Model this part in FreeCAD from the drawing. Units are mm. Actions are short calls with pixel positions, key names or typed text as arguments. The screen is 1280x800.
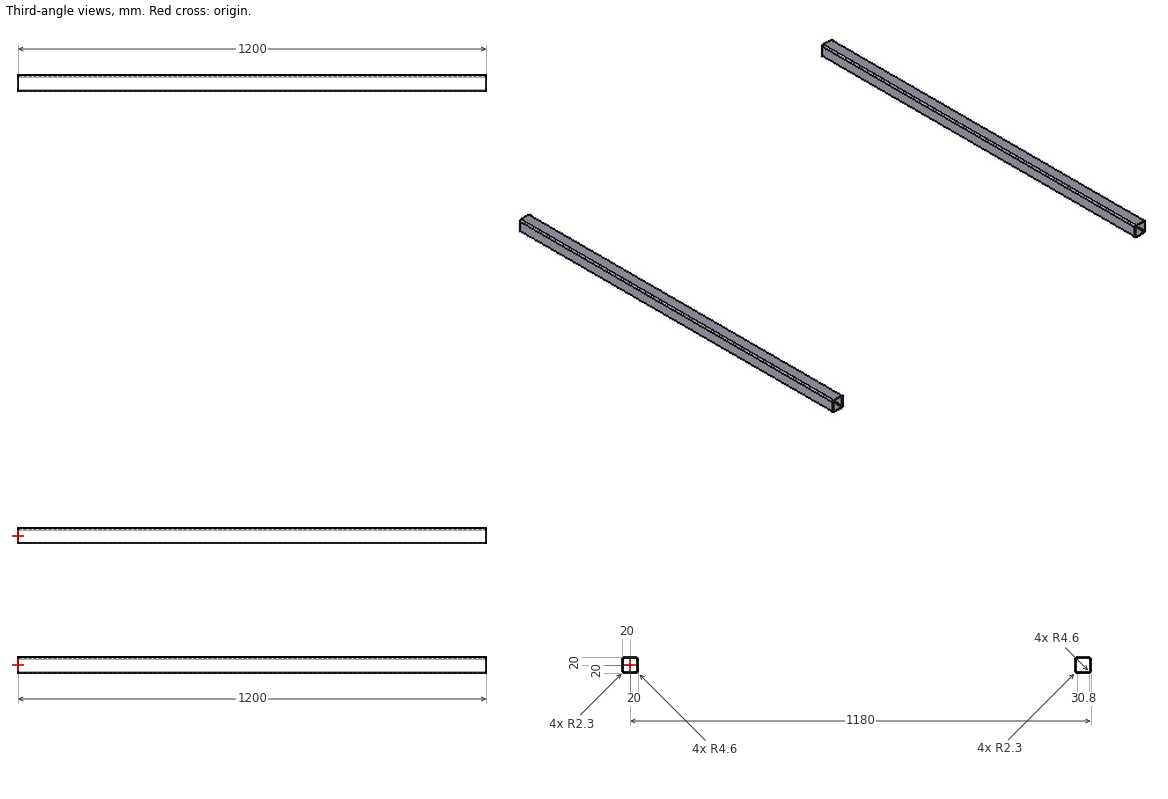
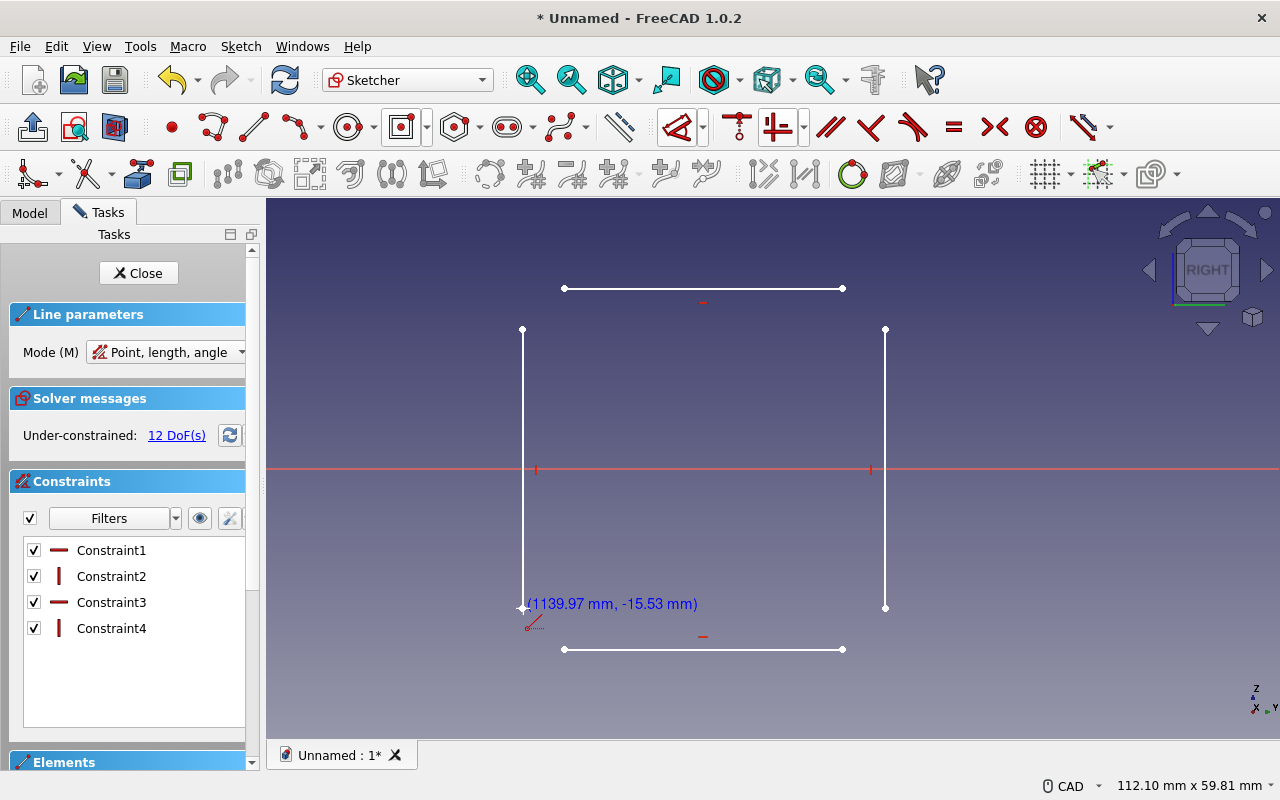
click(294, 128)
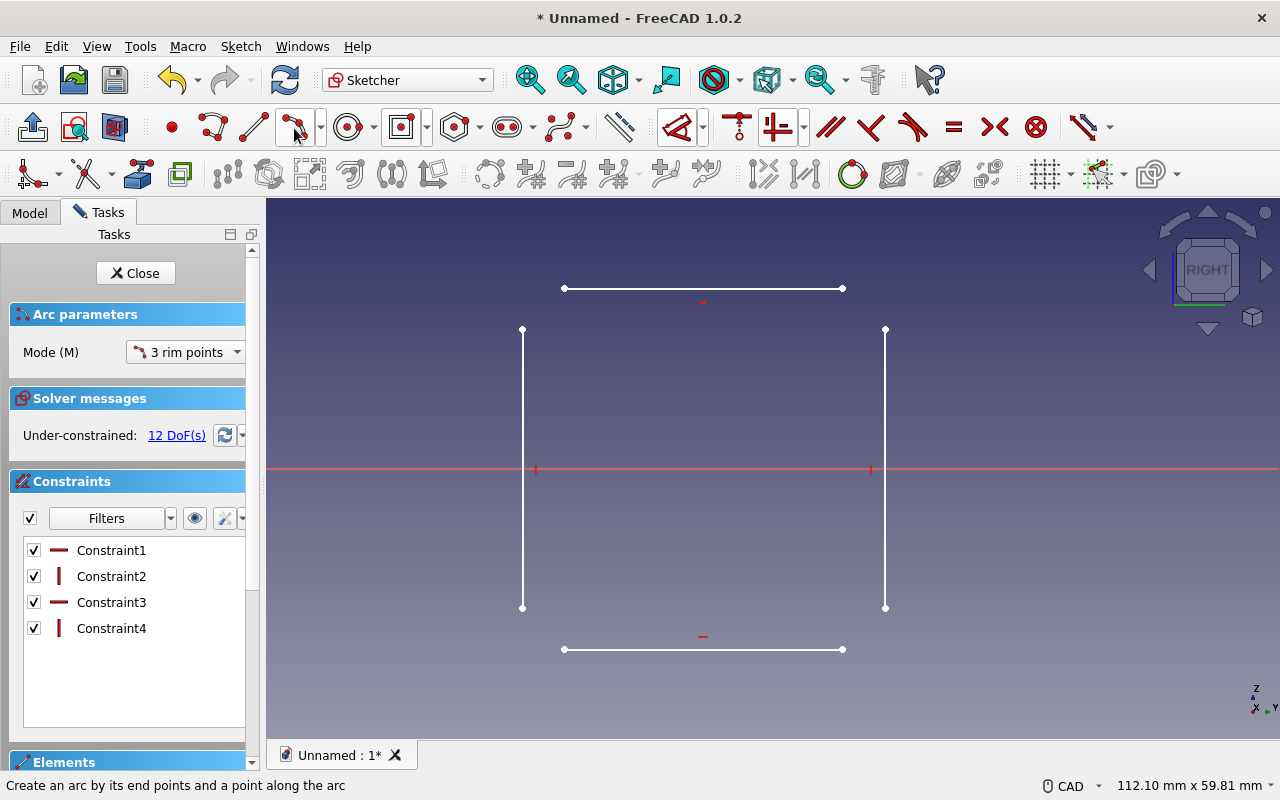
click(843, 650)
click(885, 609)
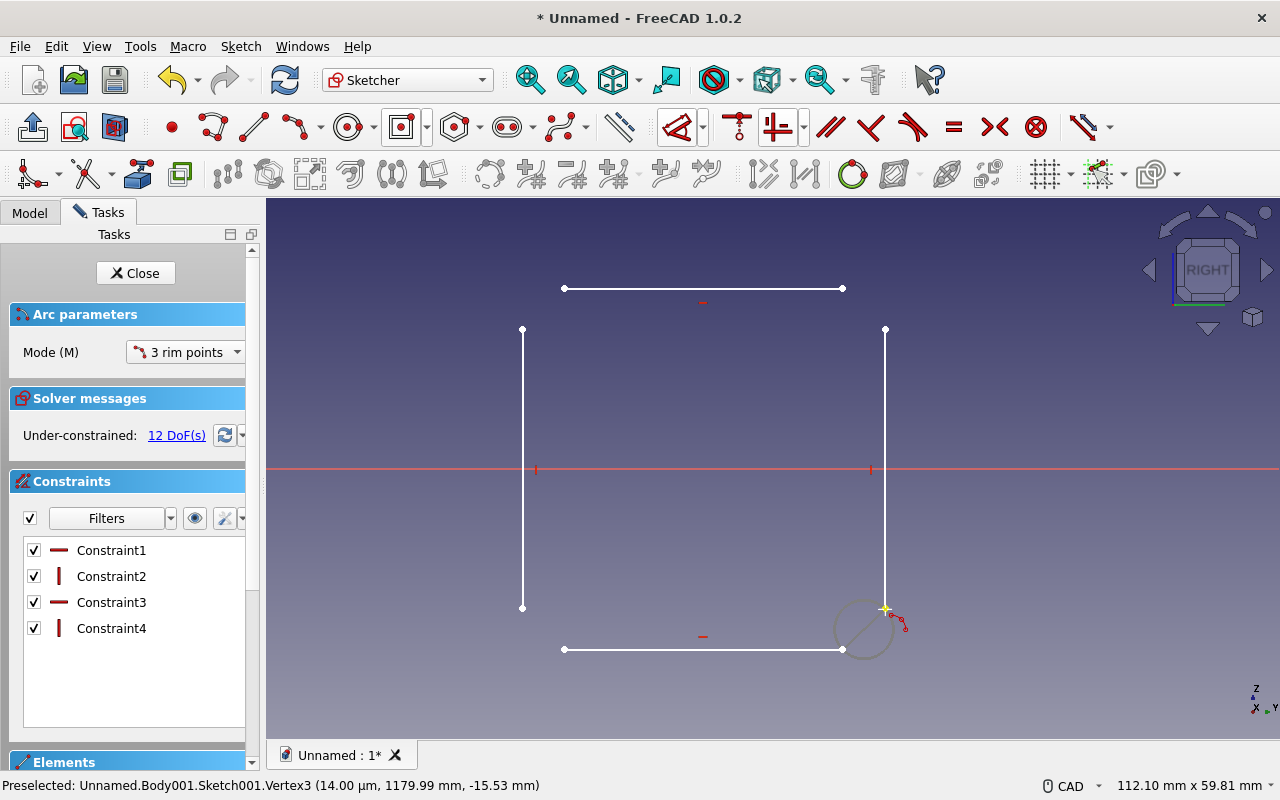
scroll(873, 637, up, 2)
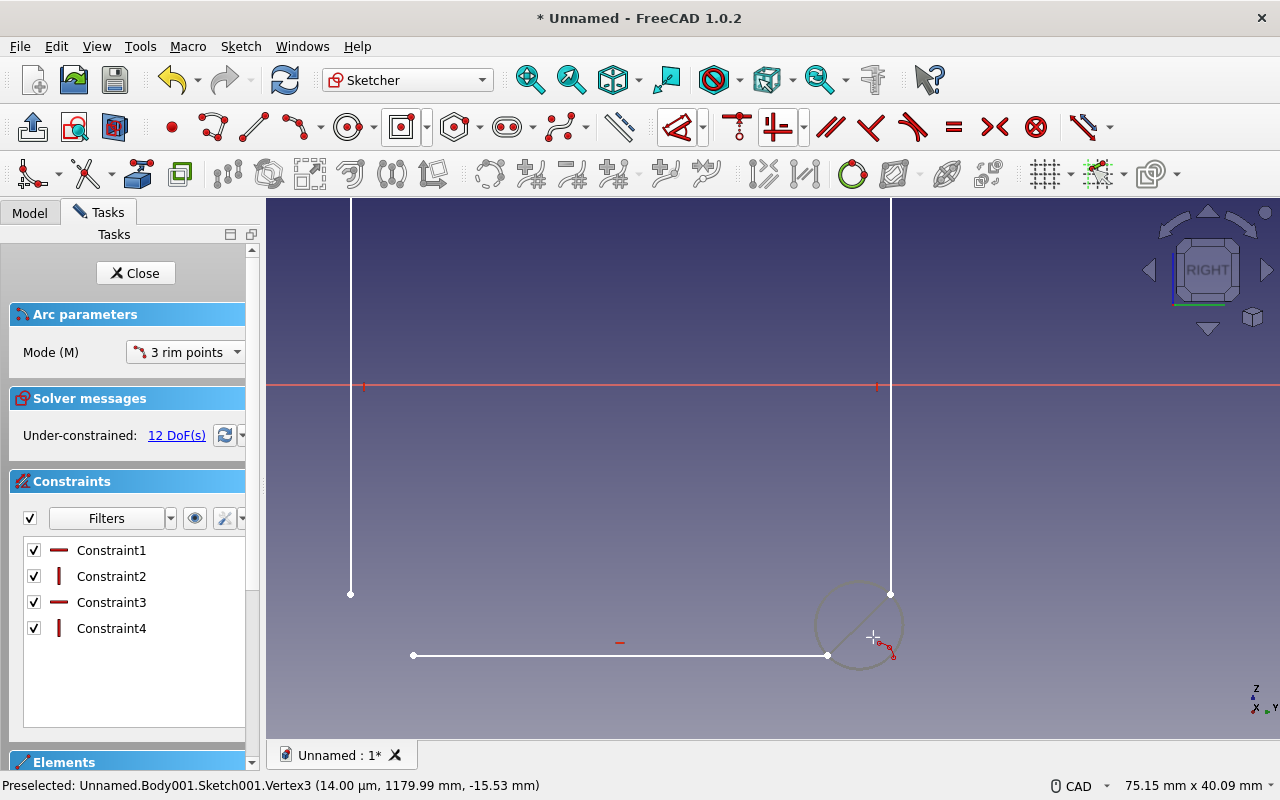
click(873, 637)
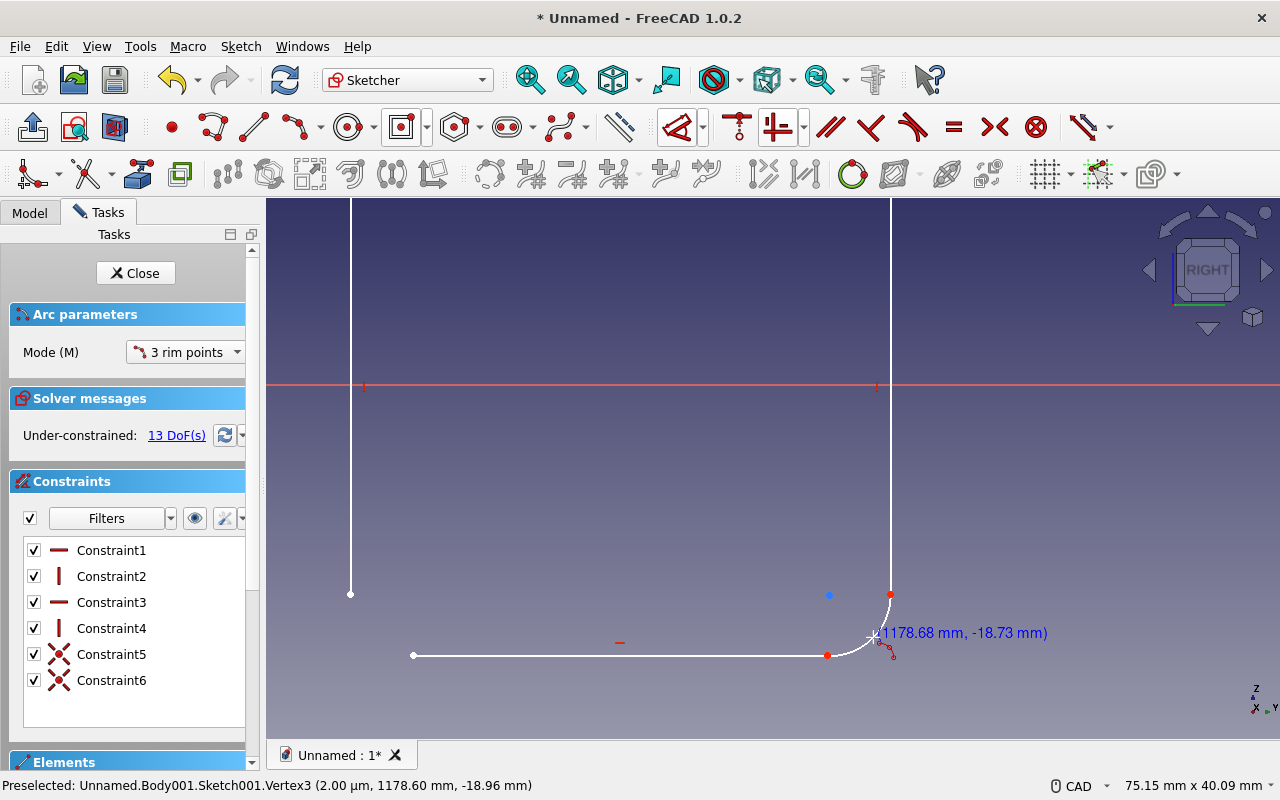
scroll(874, 638, down, 2)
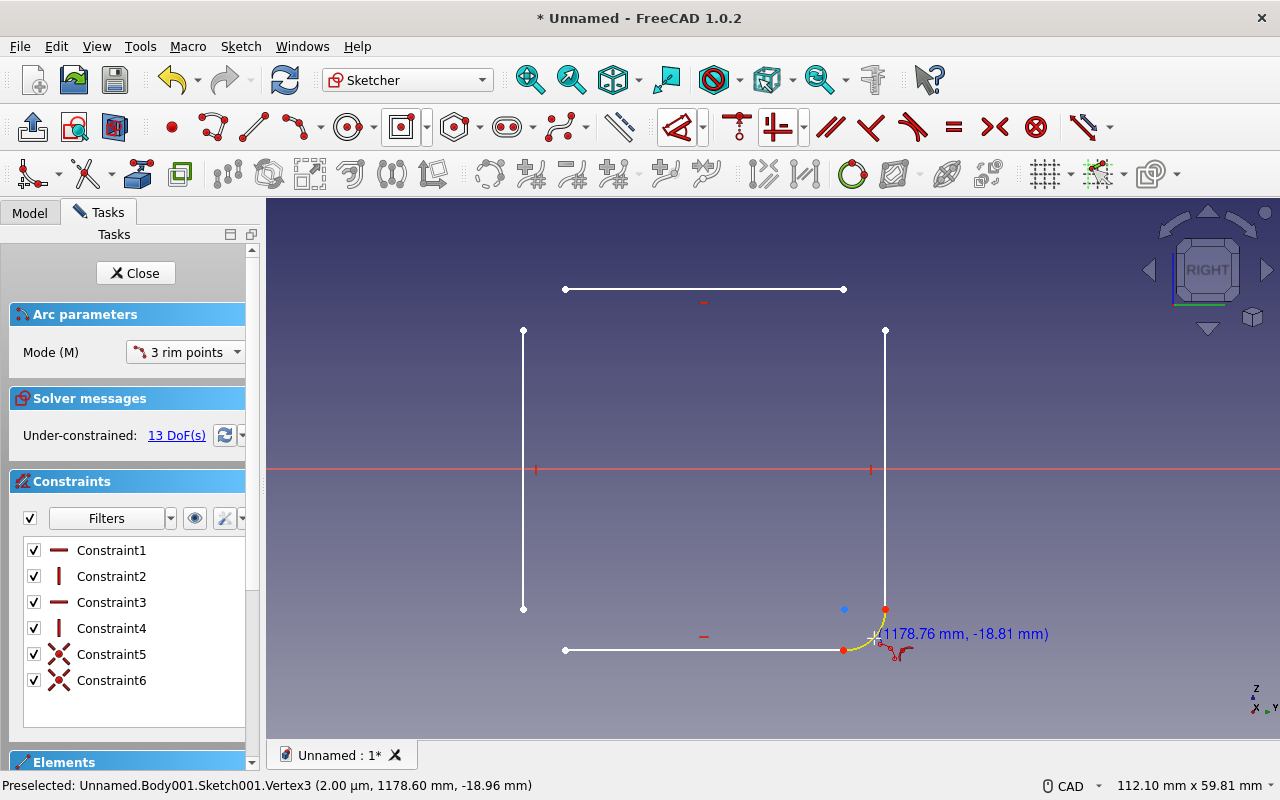
click(885, 330)
click(843, 289)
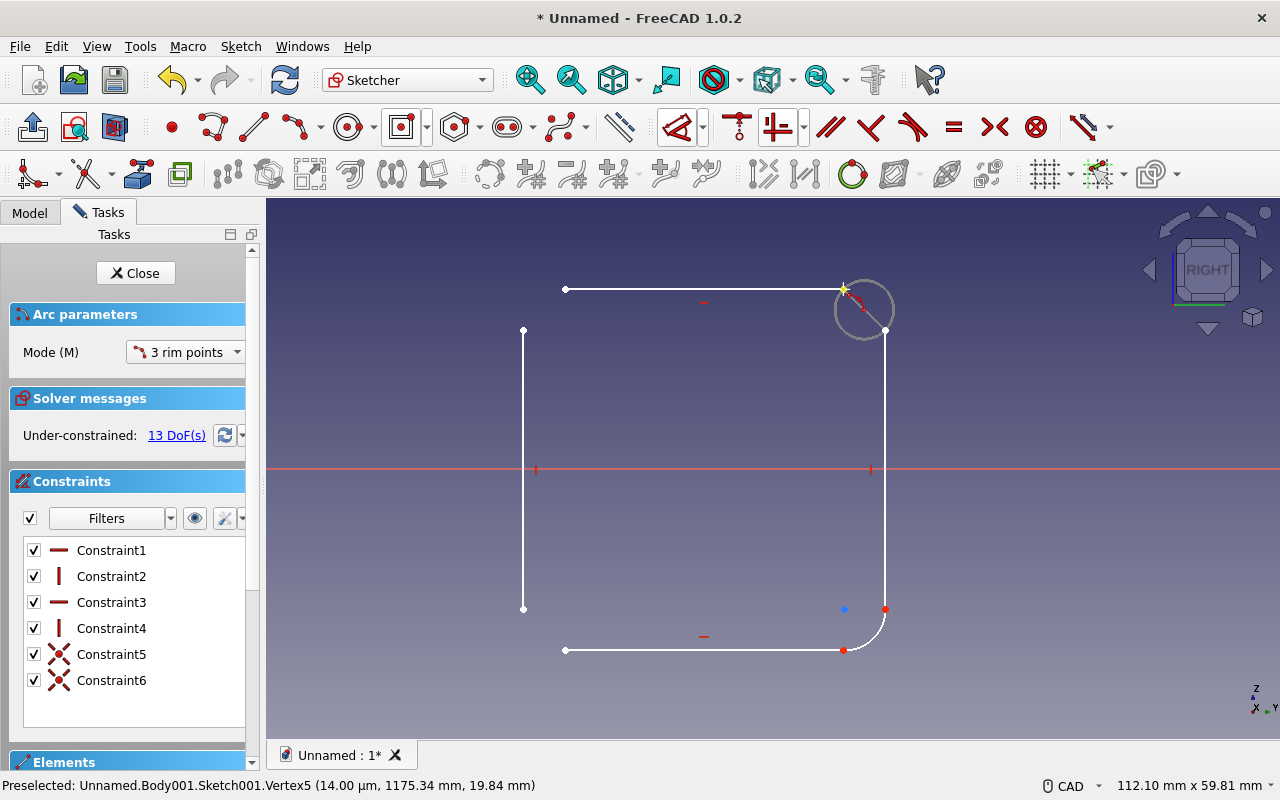
scroll(873, 300, up, 2)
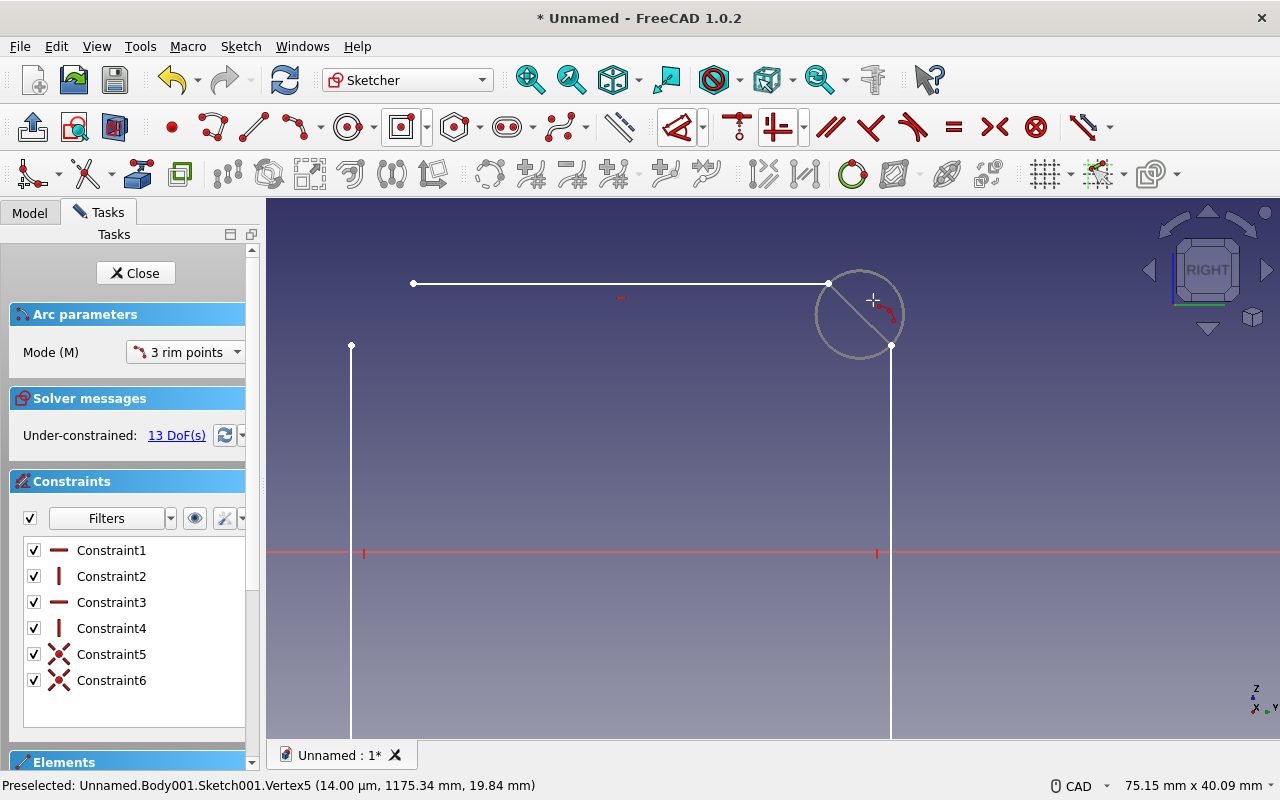
click(873, 300)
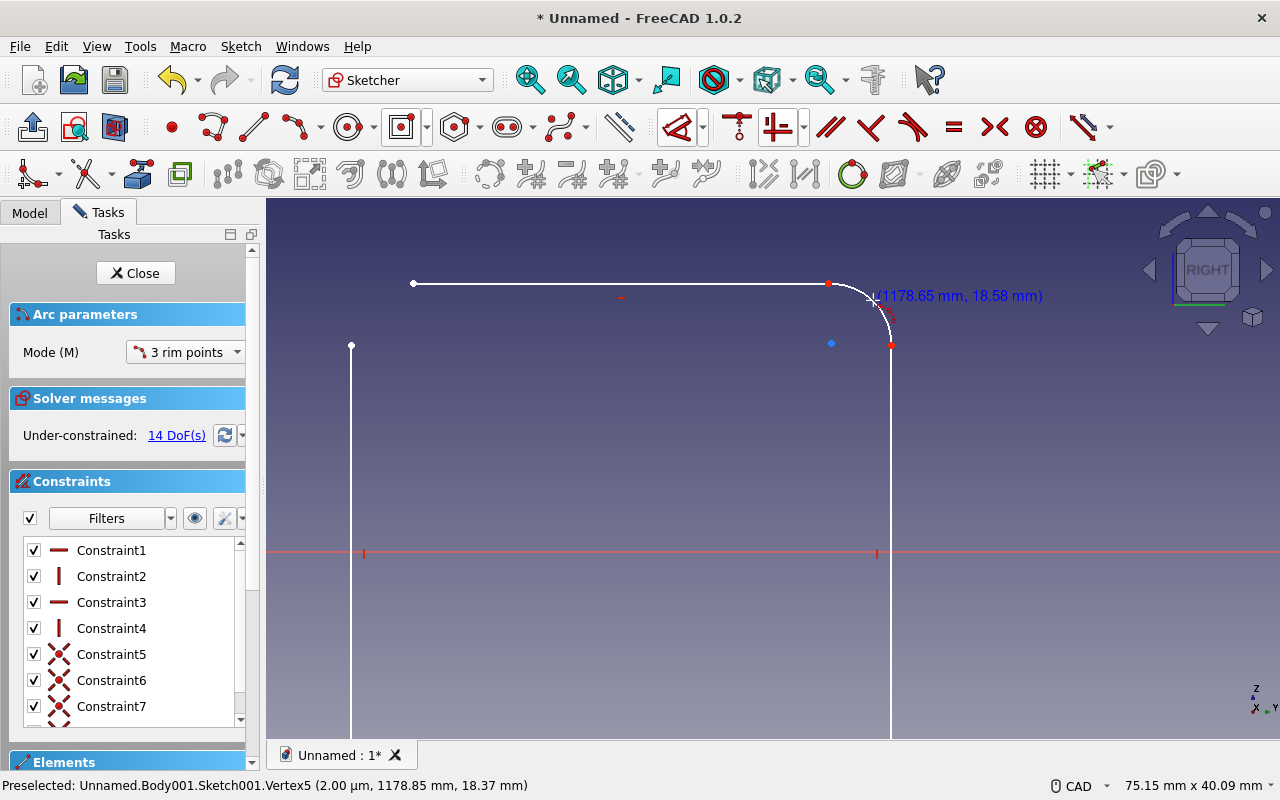
click(414, 284)
click(351, 345)
click(370, 300)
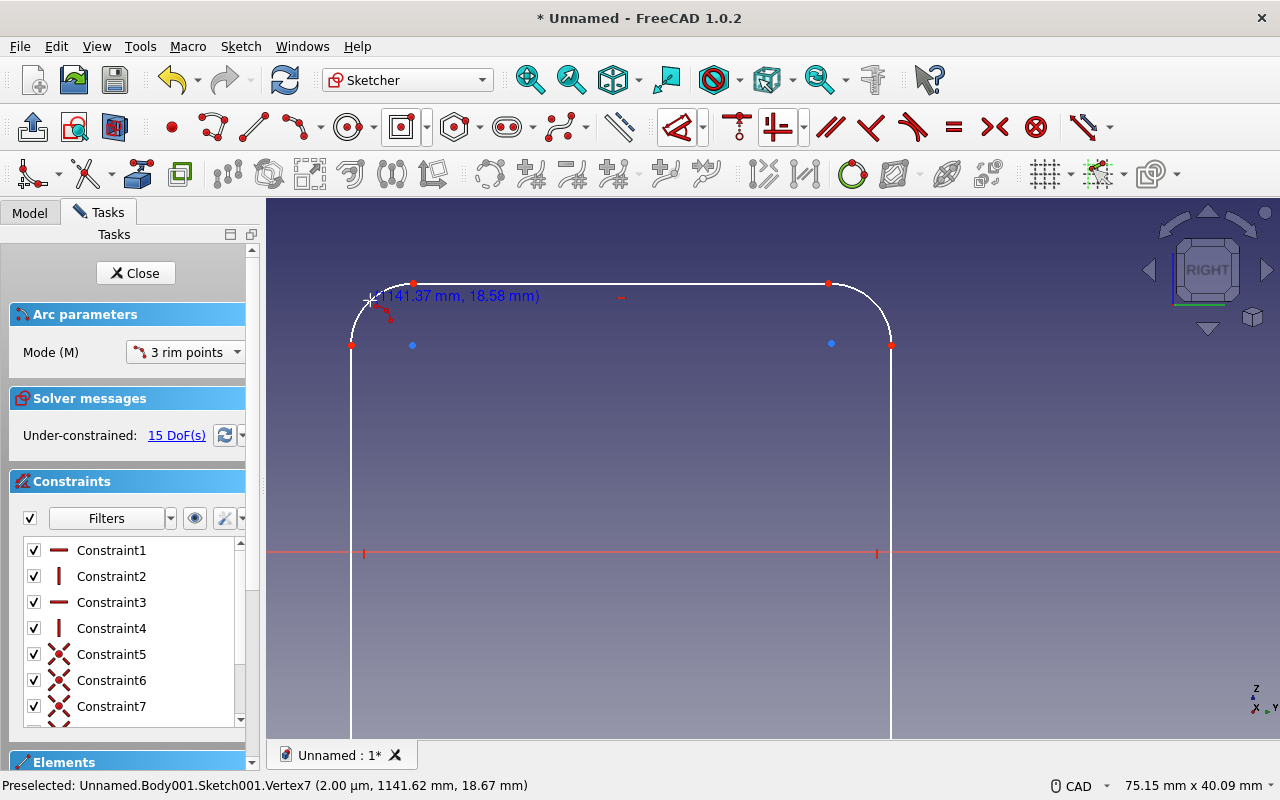
scroll(873, 299, down, 2)